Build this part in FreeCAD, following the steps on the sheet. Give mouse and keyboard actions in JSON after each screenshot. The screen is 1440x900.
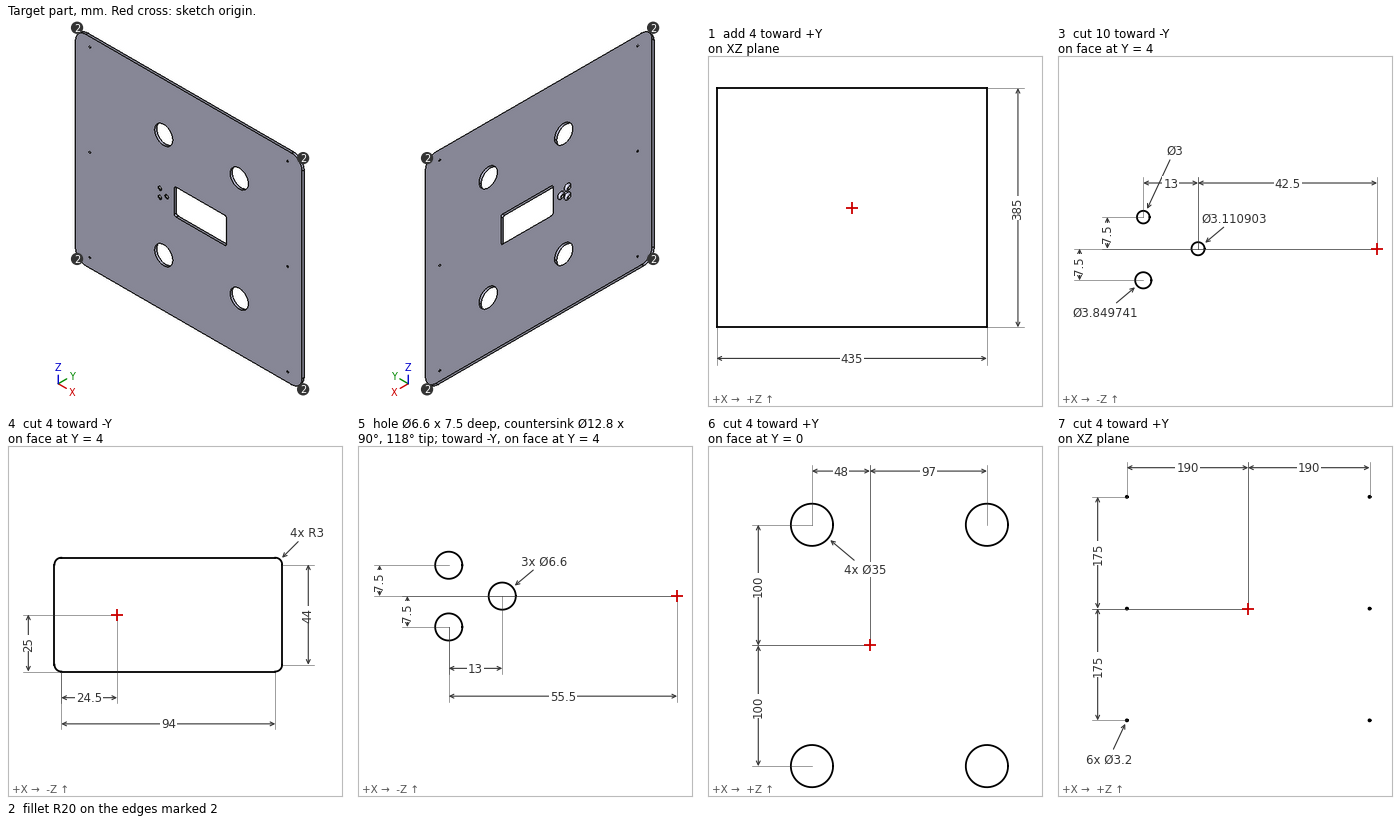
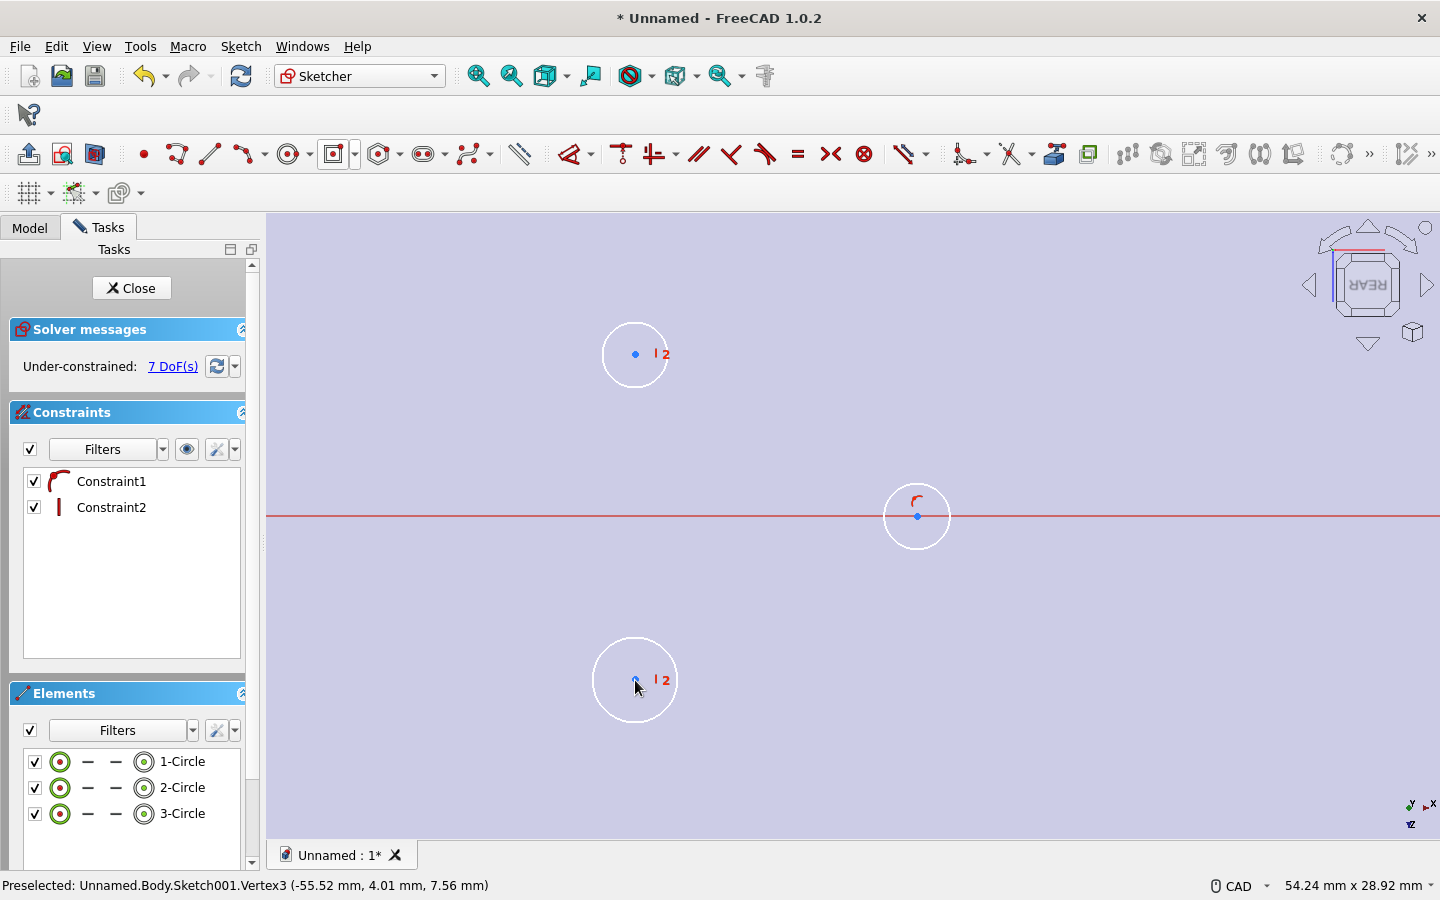
{"action": "left_click", "coordinate": [568, 154]}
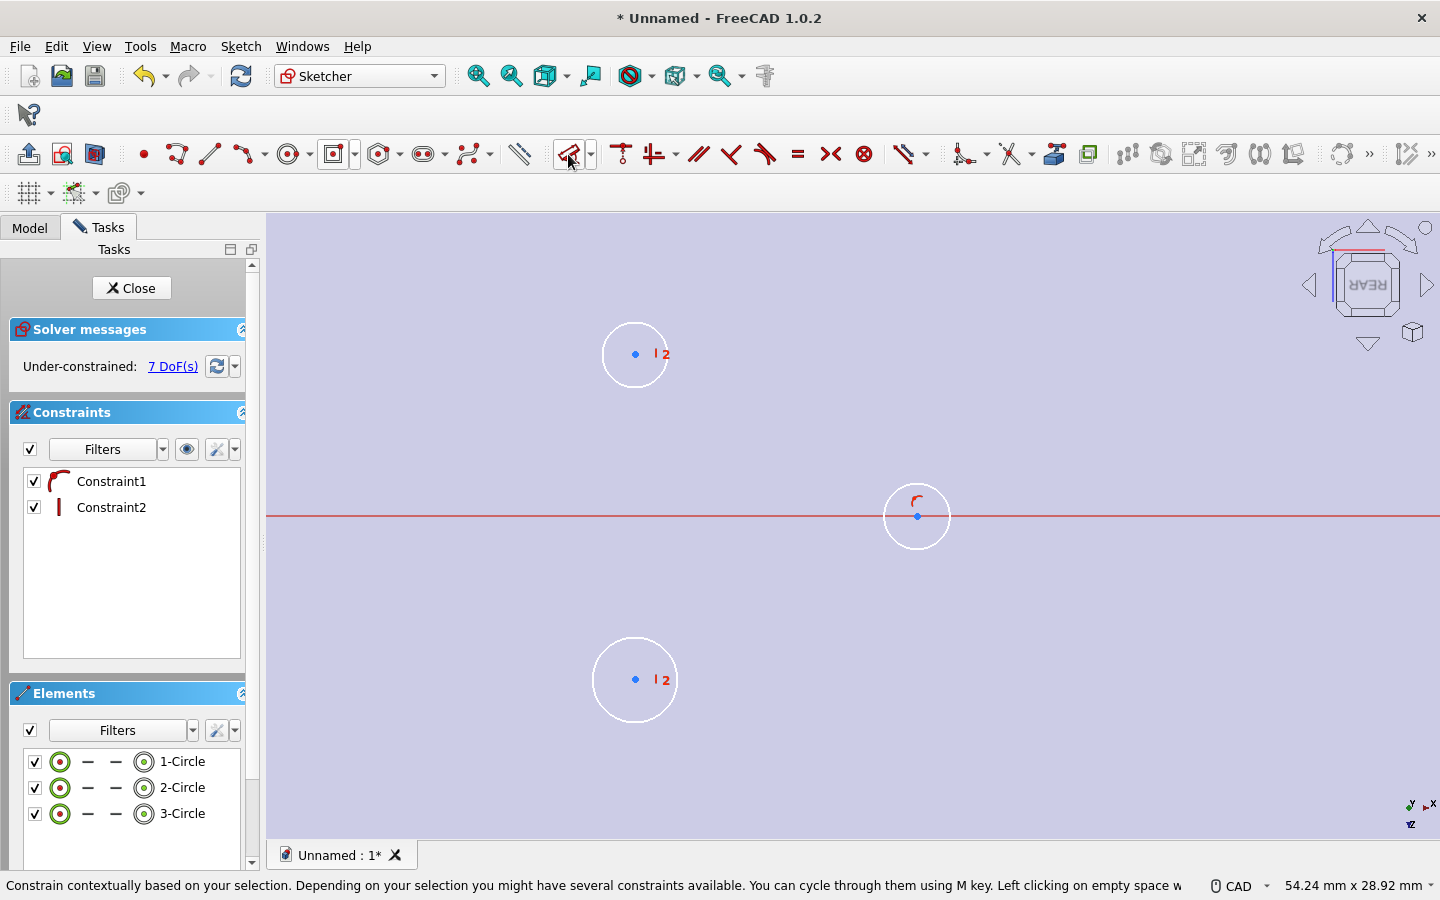
{"action": "left_click", "coordinate": [940, 493]}
{"action": "left_click", "coordinate": [962, 470]}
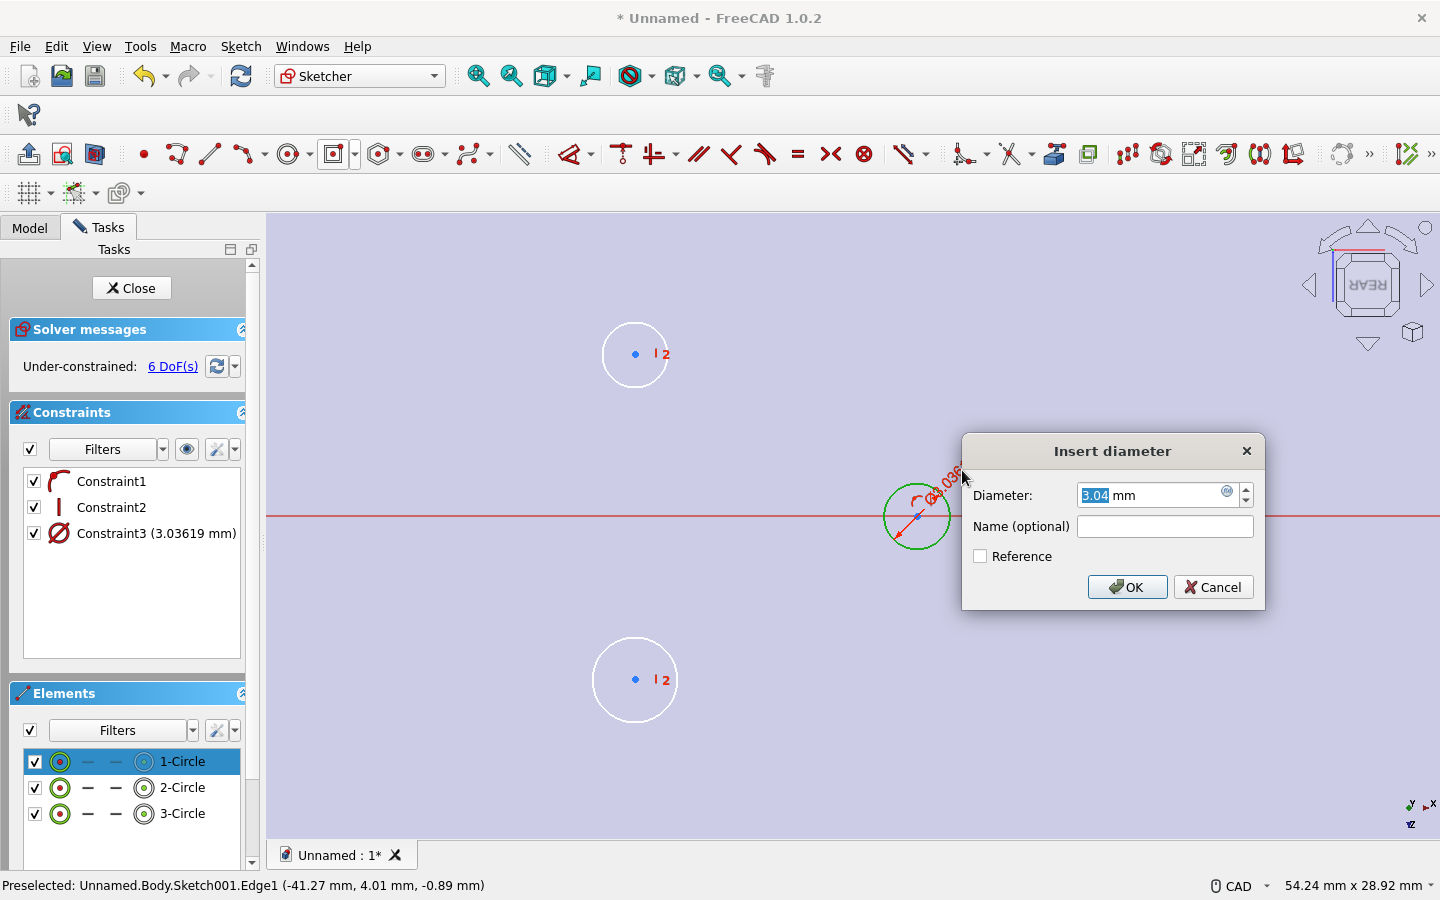
{"action": "type", "text": "3.110903"}
{"action": "key", "text": "Return"}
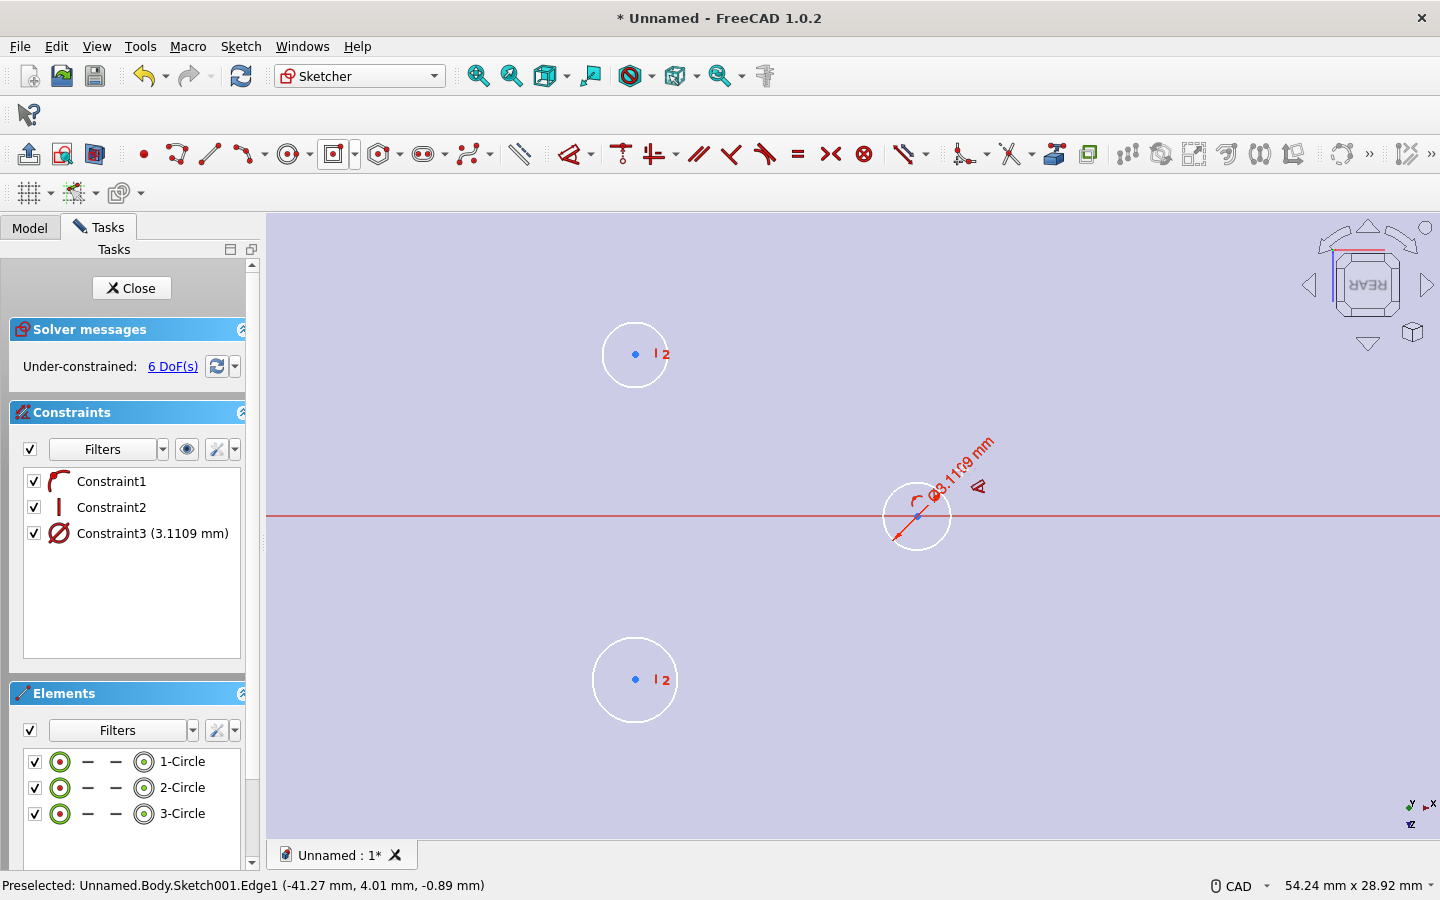
{"action": "left_click", "coordinate": [658, 332]}
{"action": "left_click", "coordinate": [681, 309]}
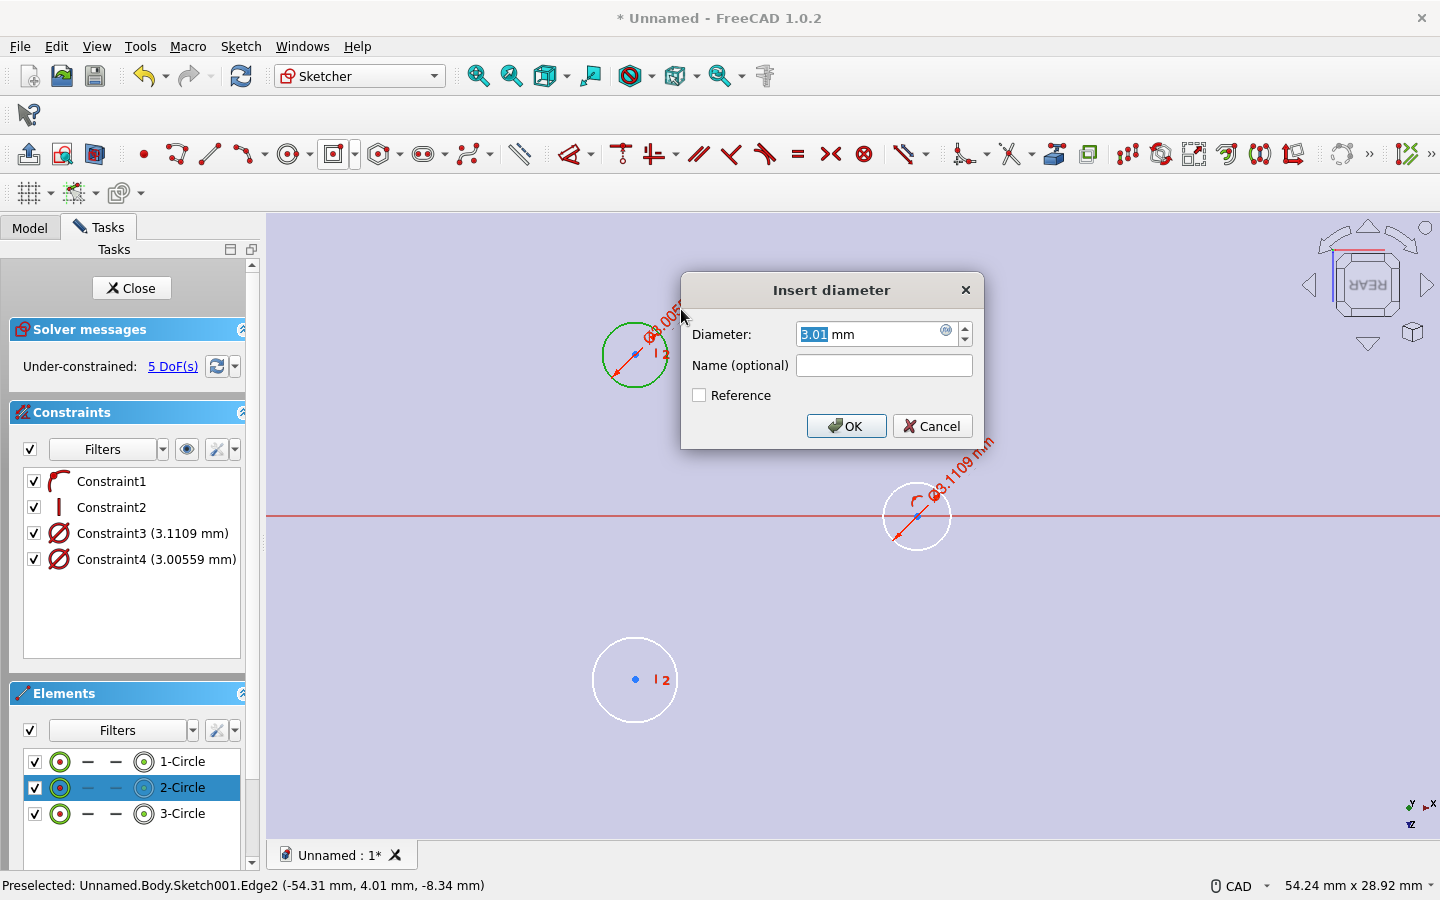
{"action": "type", "text": "3"}
{"action": "key", "text": "Return"}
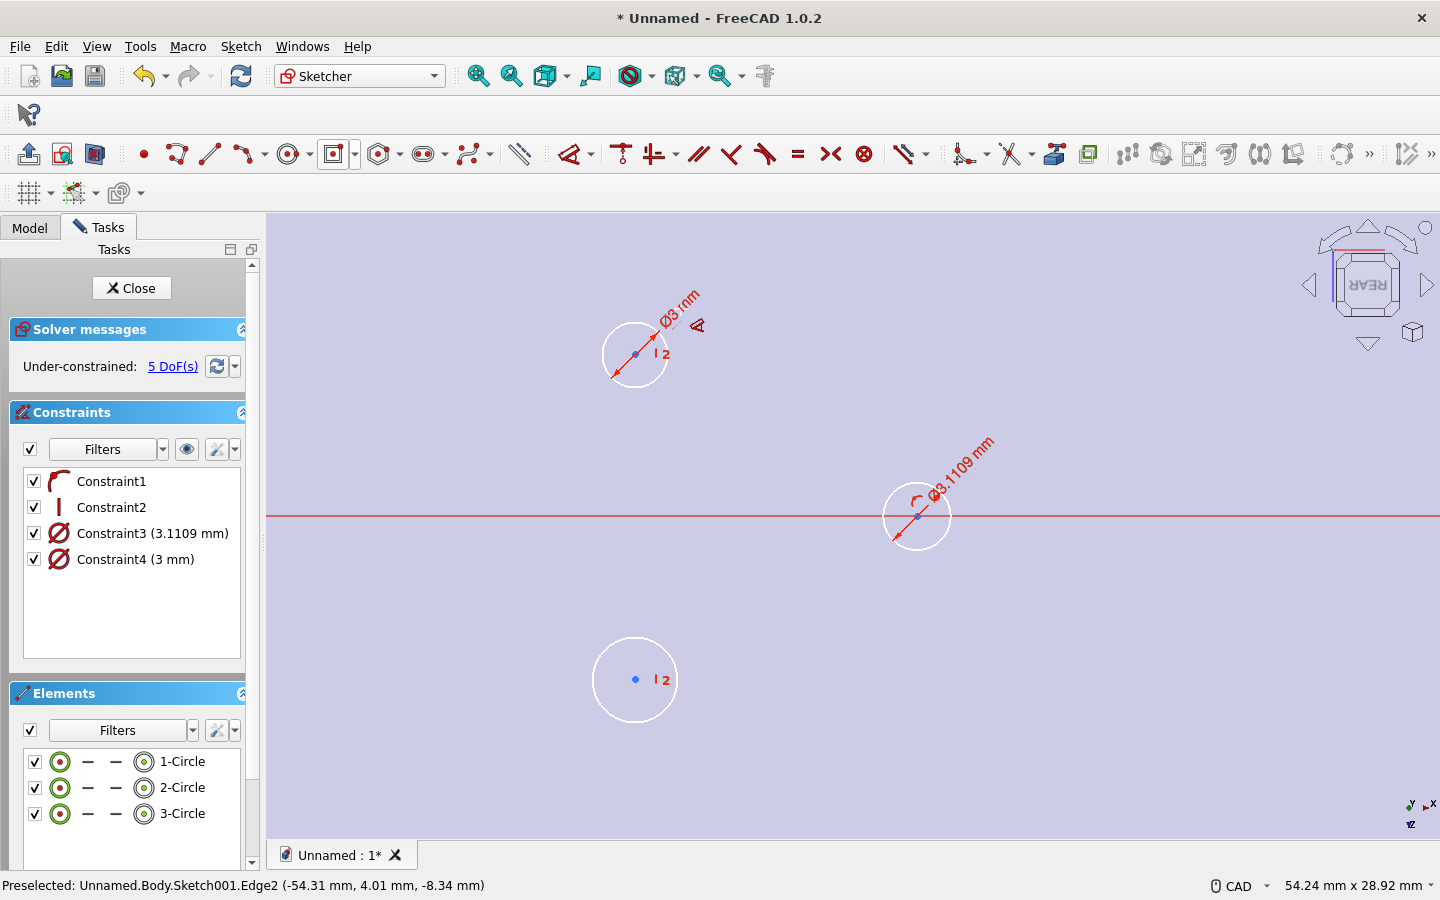
{"action": "left_click", "coordinate": [665, 650]}
{"action": "left_click", "coordinate": [688, 627]}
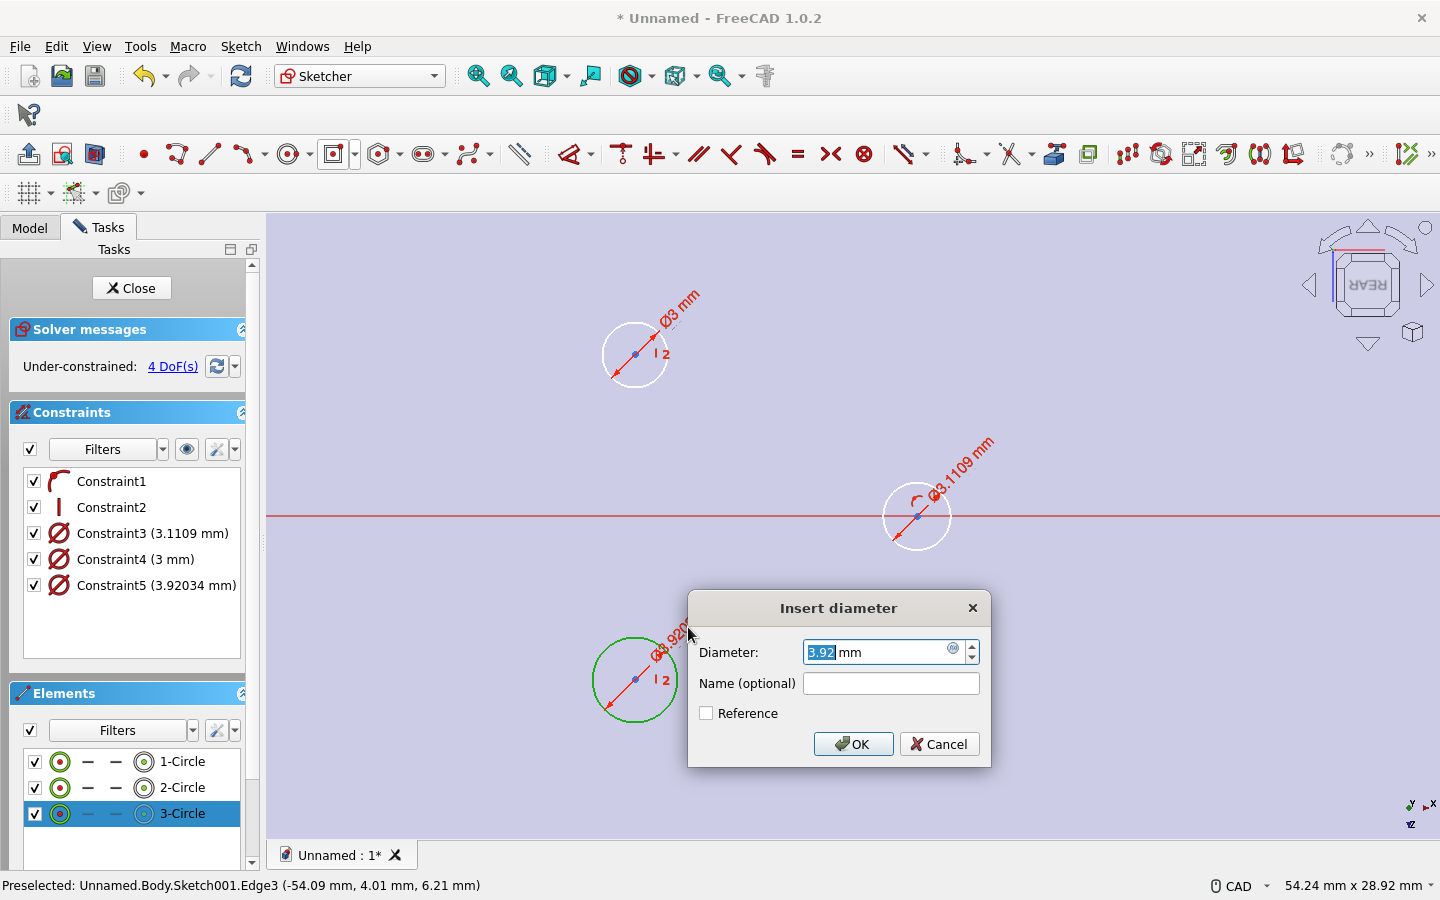
{"action": "type", "text": "3.849741"}
{"action": "key", "text": "Return"}